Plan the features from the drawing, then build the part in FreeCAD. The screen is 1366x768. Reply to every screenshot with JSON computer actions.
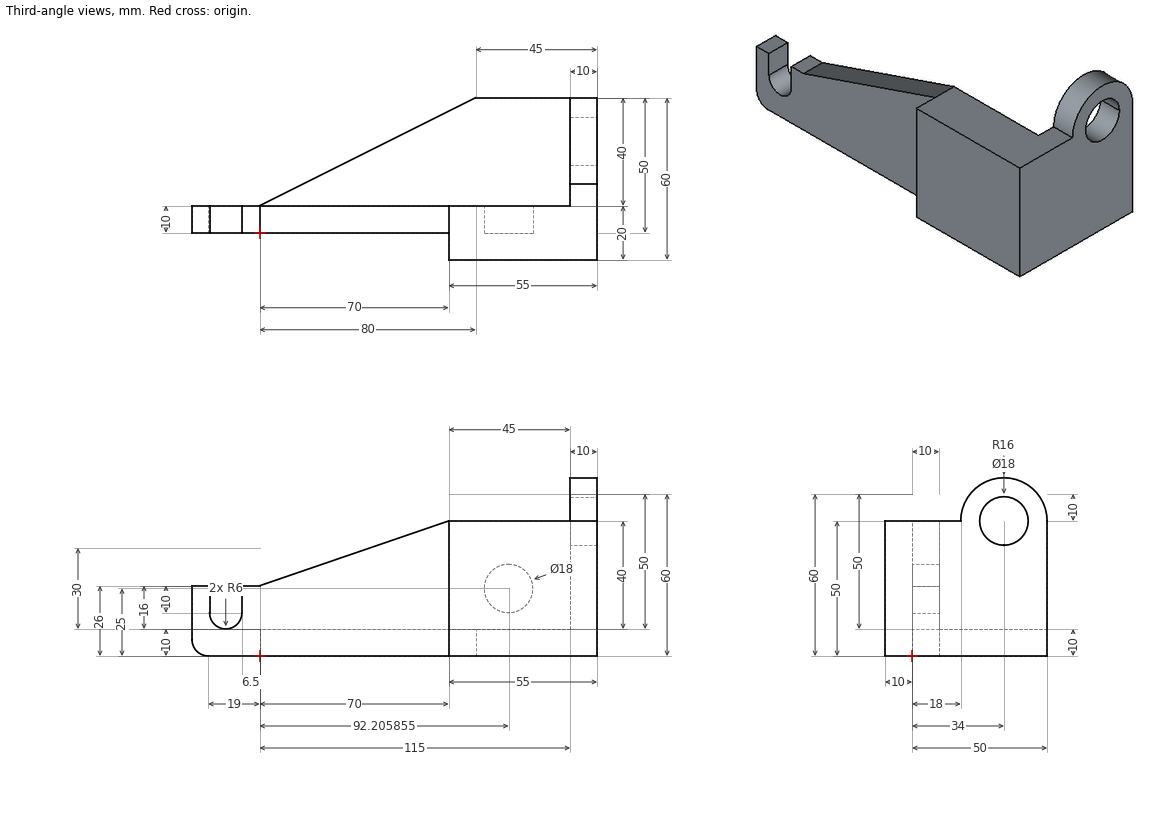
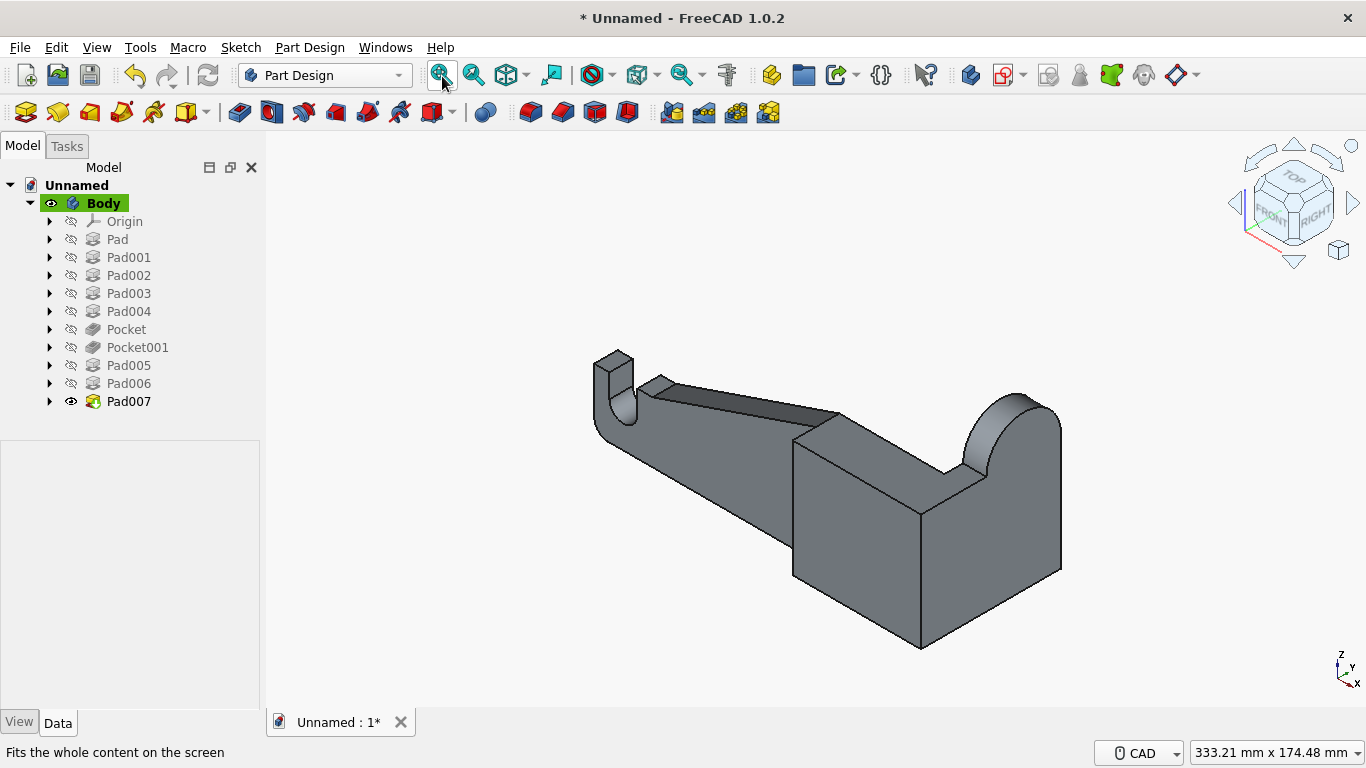
{"action": "left_click", "coordinate": [991, 544]}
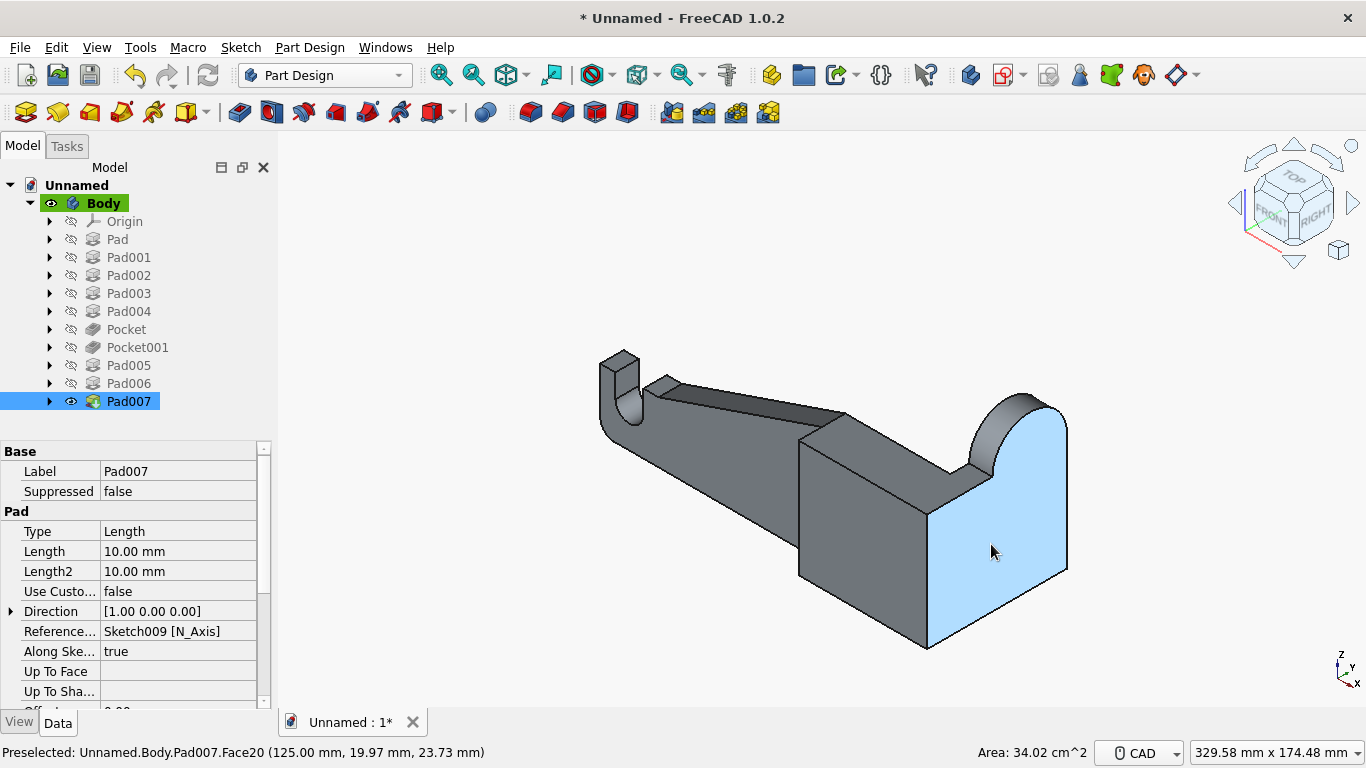
{"action": "left_click", "coordinate": [1004, 76]}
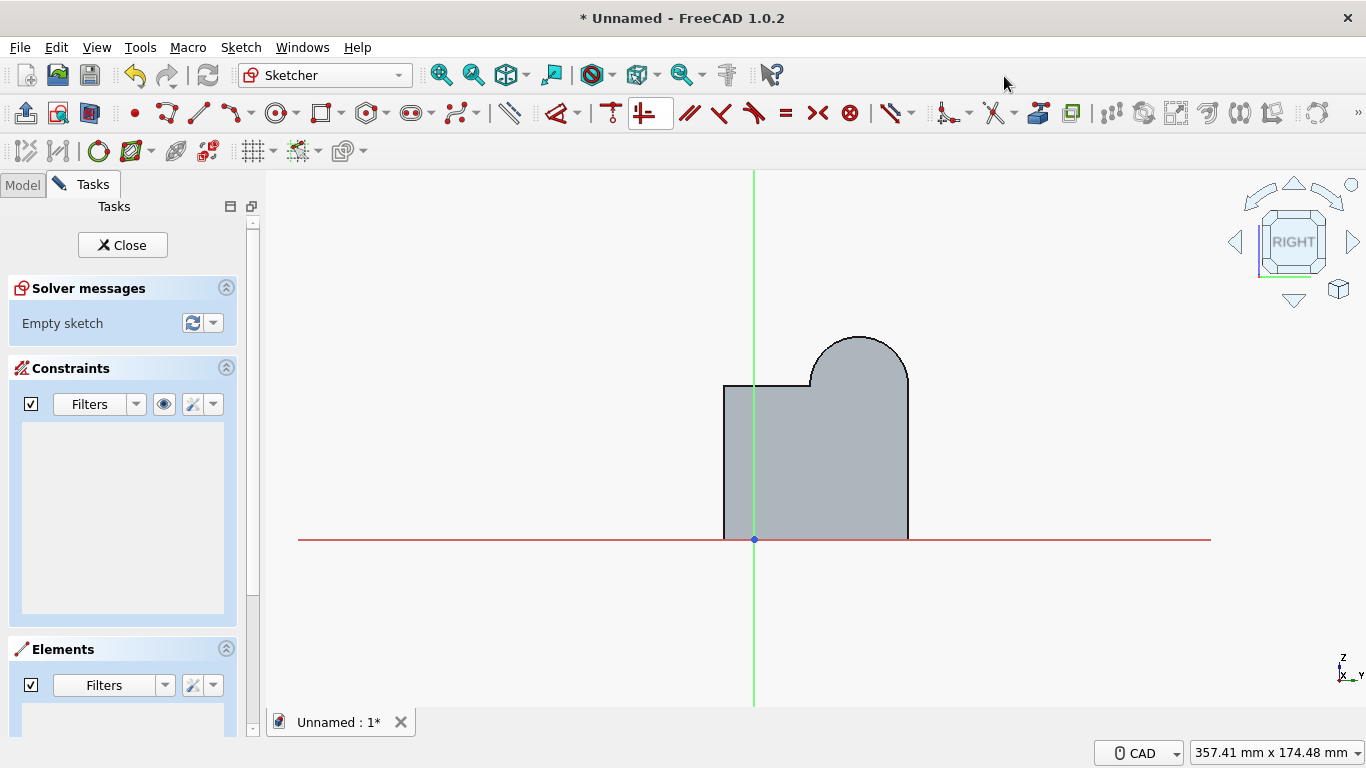
{"action": "scroll", "coordinate": [881, 376], "scroll_direction": "up", "scroll_amount": 9}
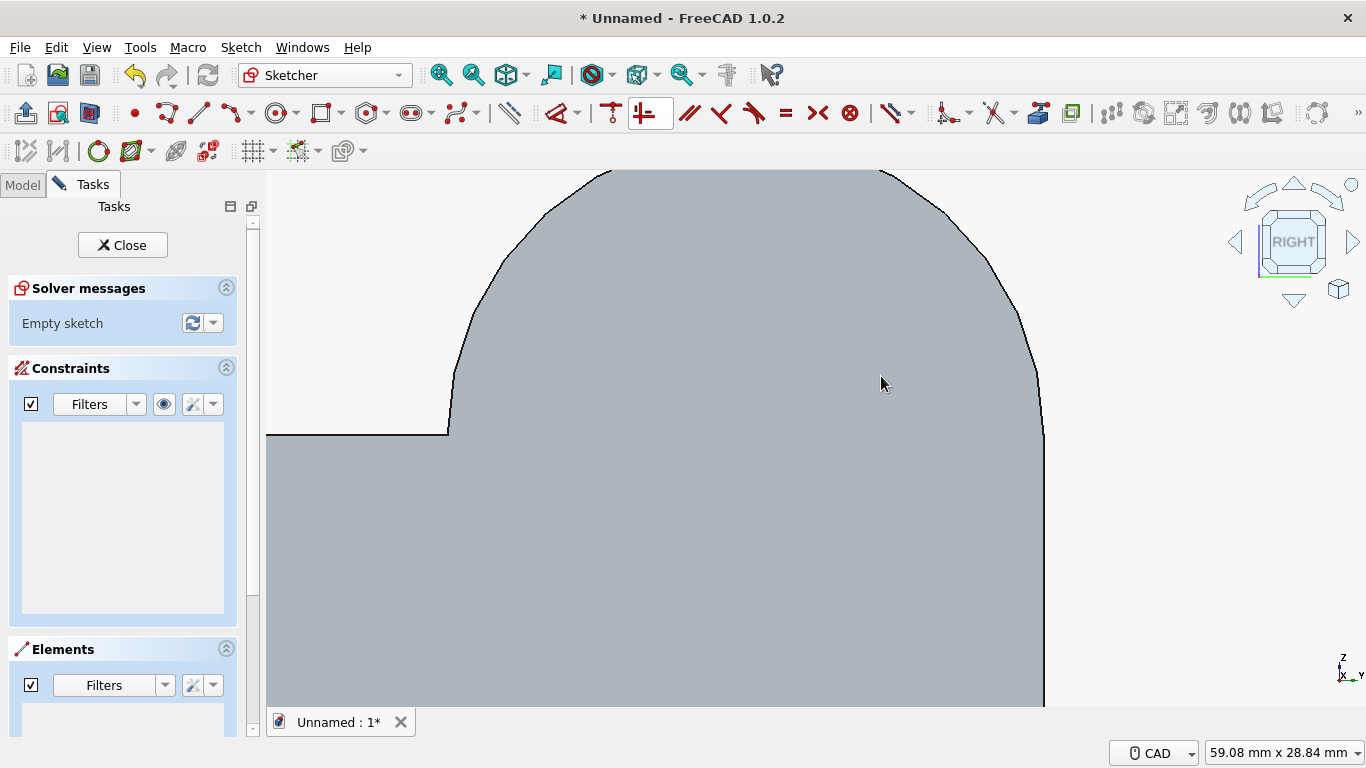
{"action": "left_click", "coordinate": [276, 114]}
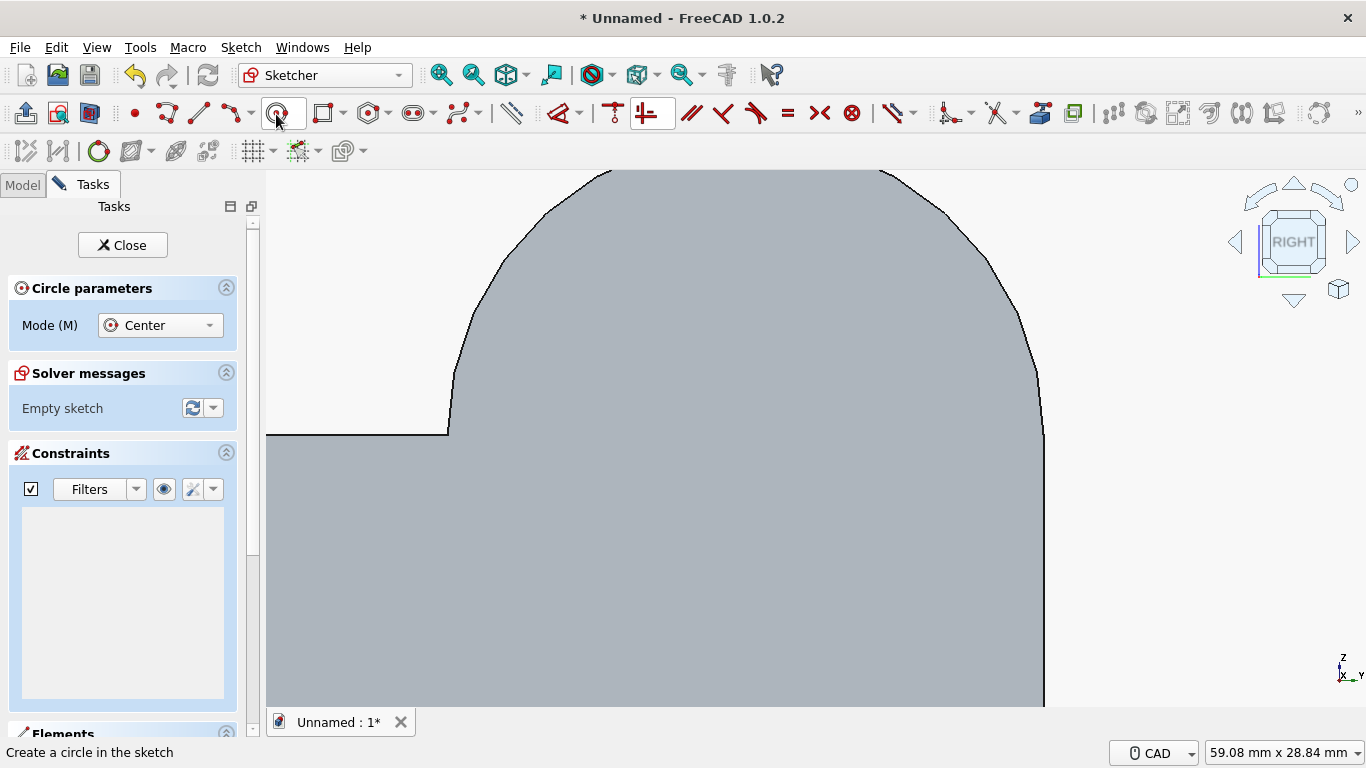
{"action": "left_click", "coordinate": [746, 435]}
{"action": "left_click", "coordinate": [864, 316]}
{"action": "key", "text": "Escape"}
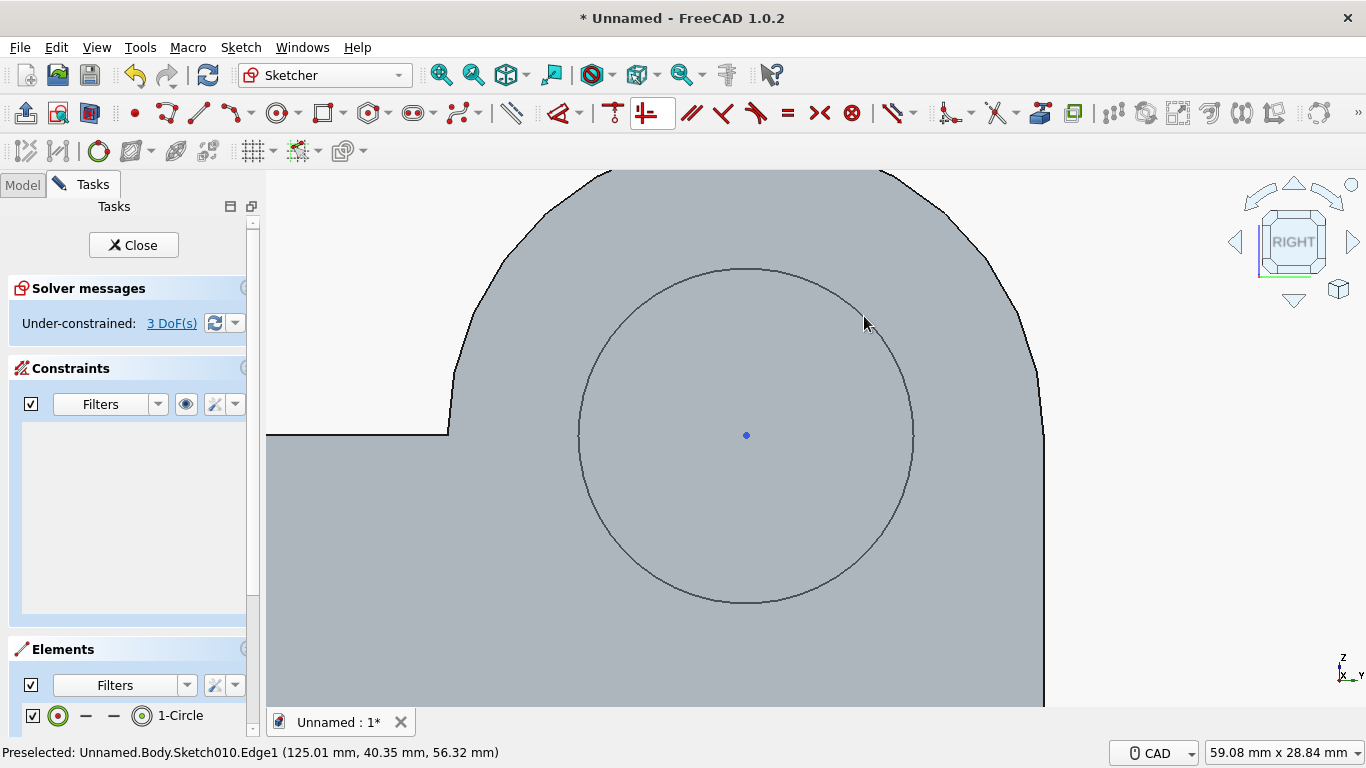
{"action": "left_click", "coordinate": [558, 114]}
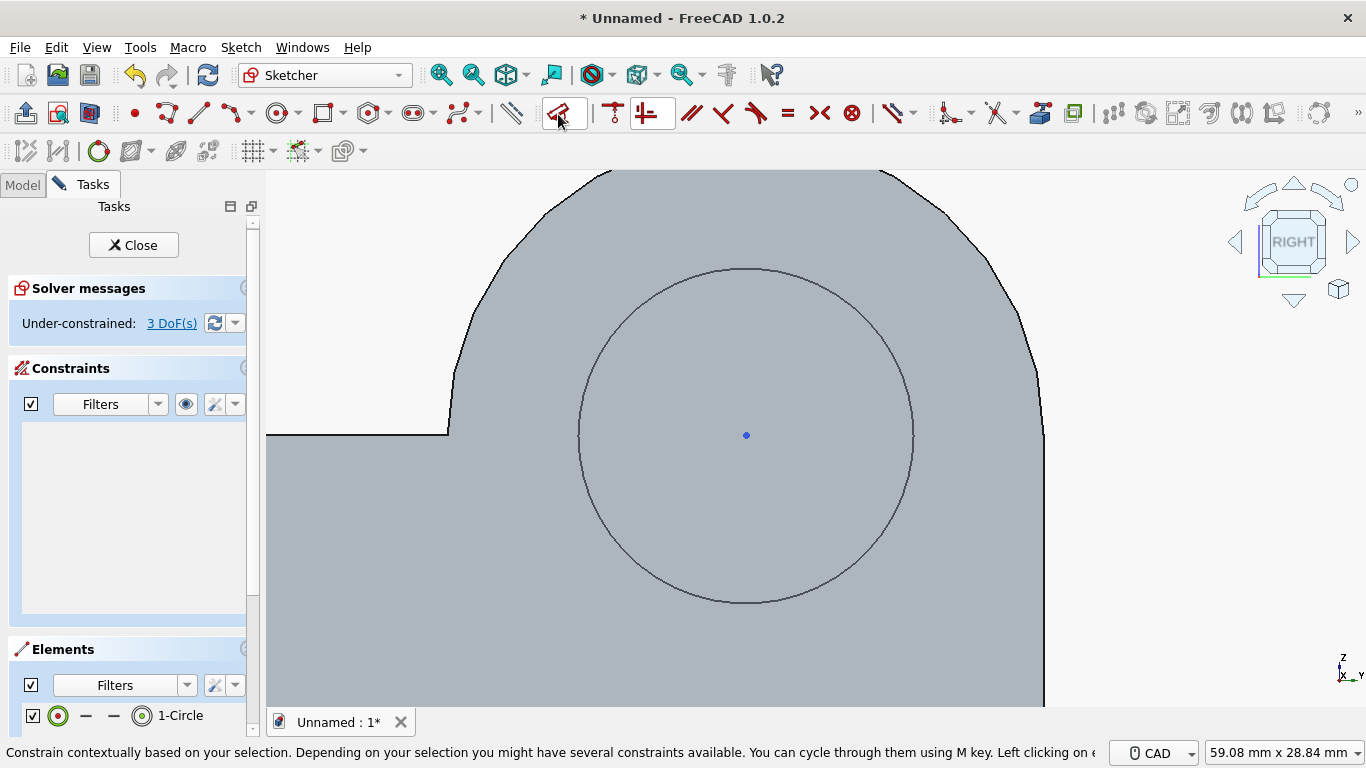
{"action": "left_click", "coordinate": [864, 317]}
{"action": "left_click", "coordinate": [887, 294]}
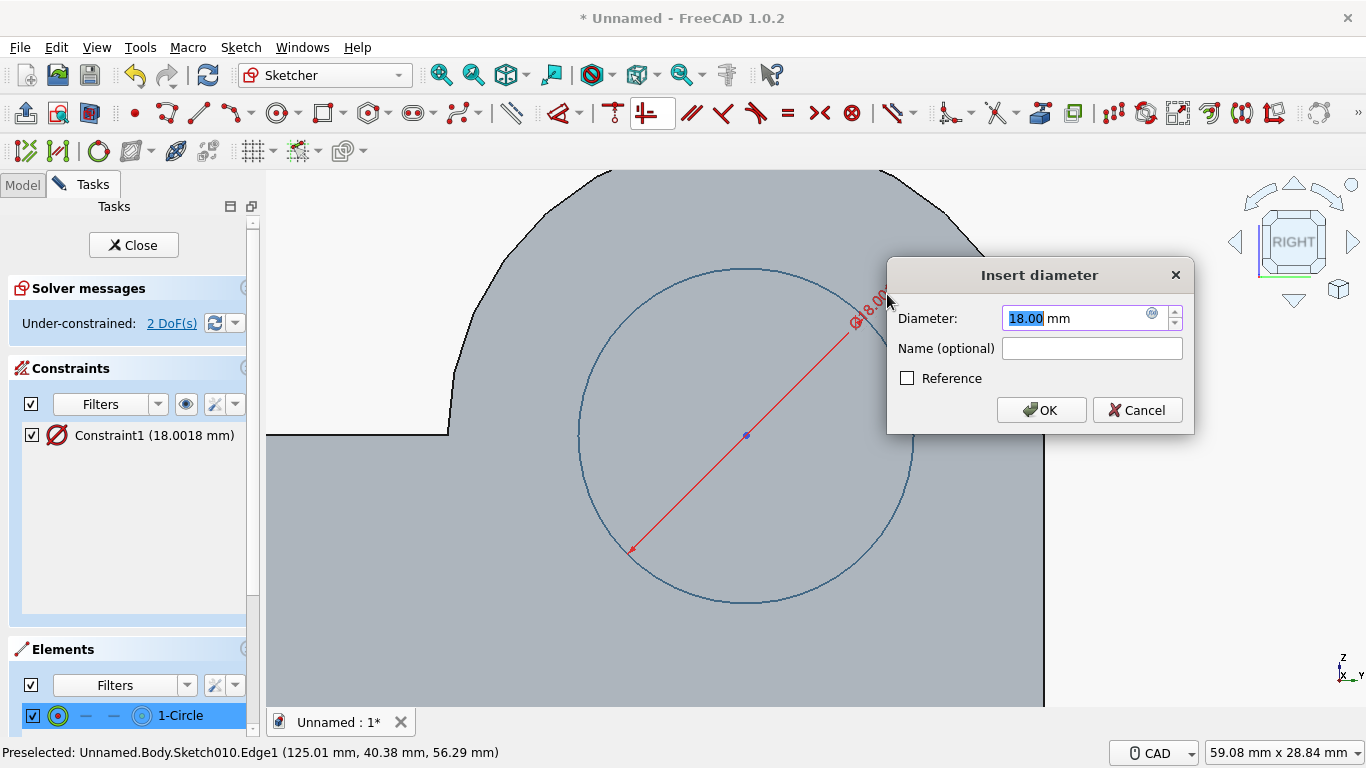
{"action": "type", "text": "18"}
{"action": "key", "text": "Return"}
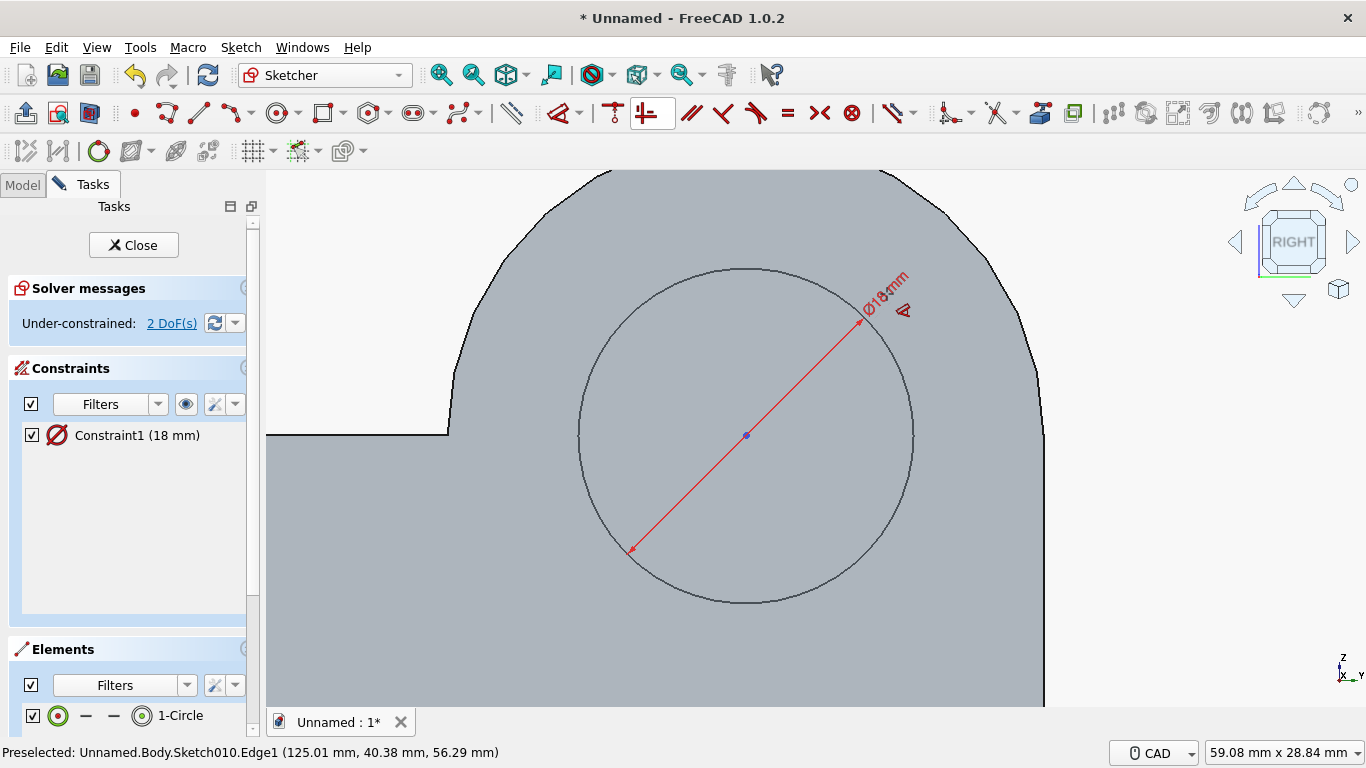
{"action": "left_click", "coordinate": [746, 436]}
{"action": "left_click", "coordinate": [520, 402]}